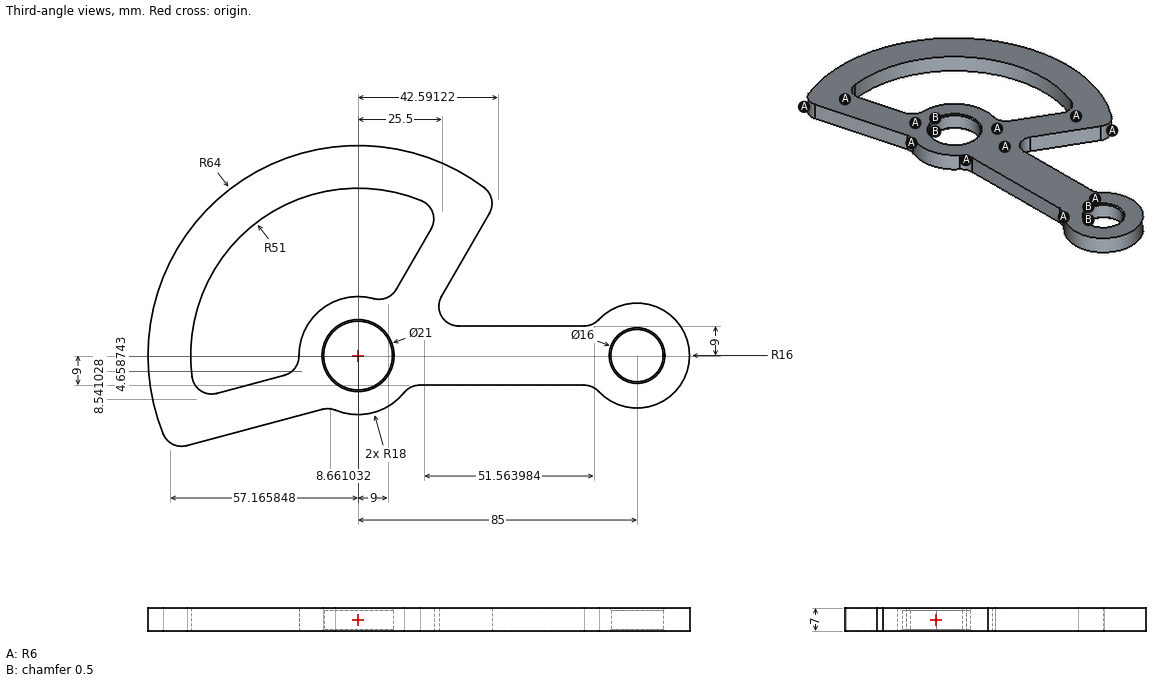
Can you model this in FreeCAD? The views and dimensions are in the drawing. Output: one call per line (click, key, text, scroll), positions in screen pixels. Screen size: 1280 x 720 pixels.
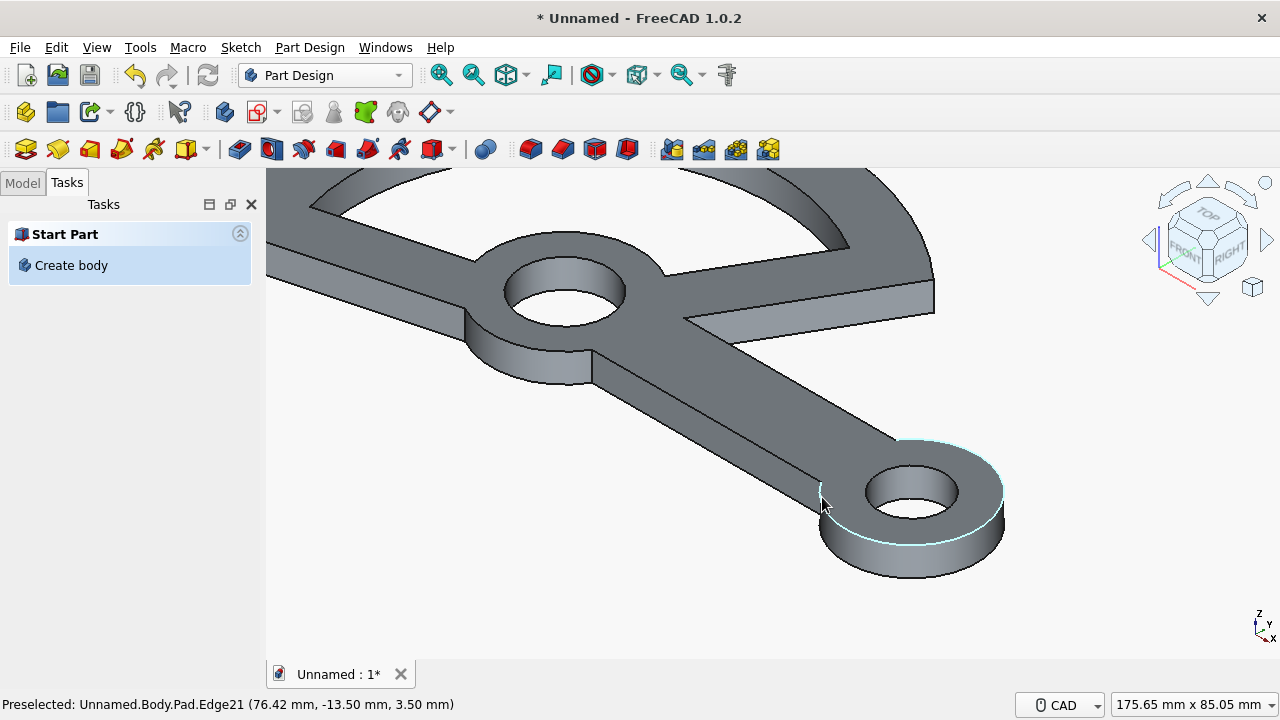
click(442, 76)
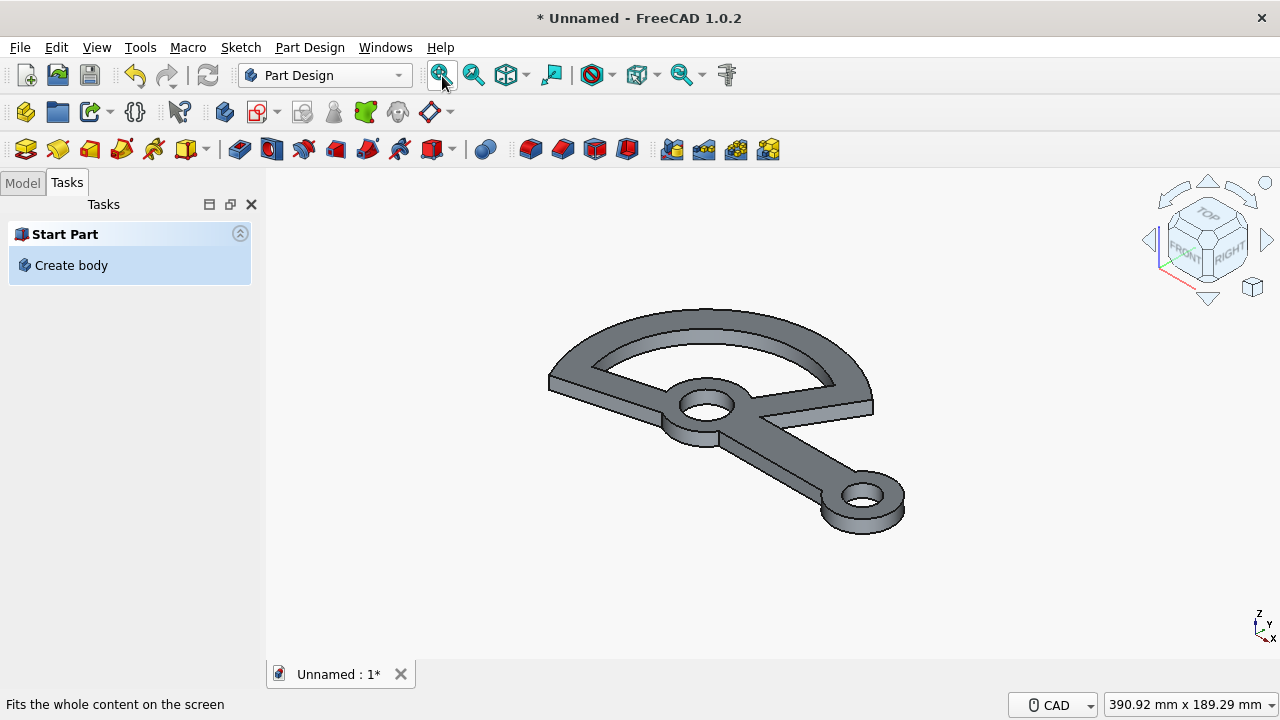
key(2)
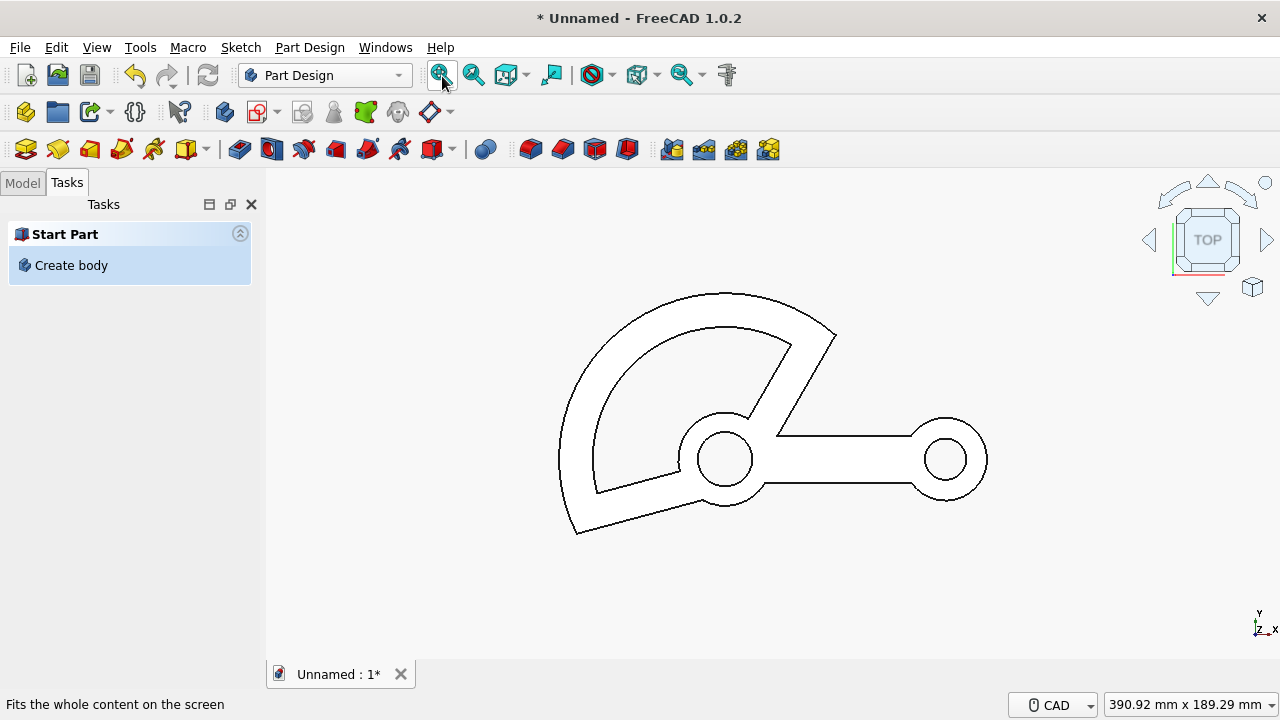
scroll(911, 482, up, 4)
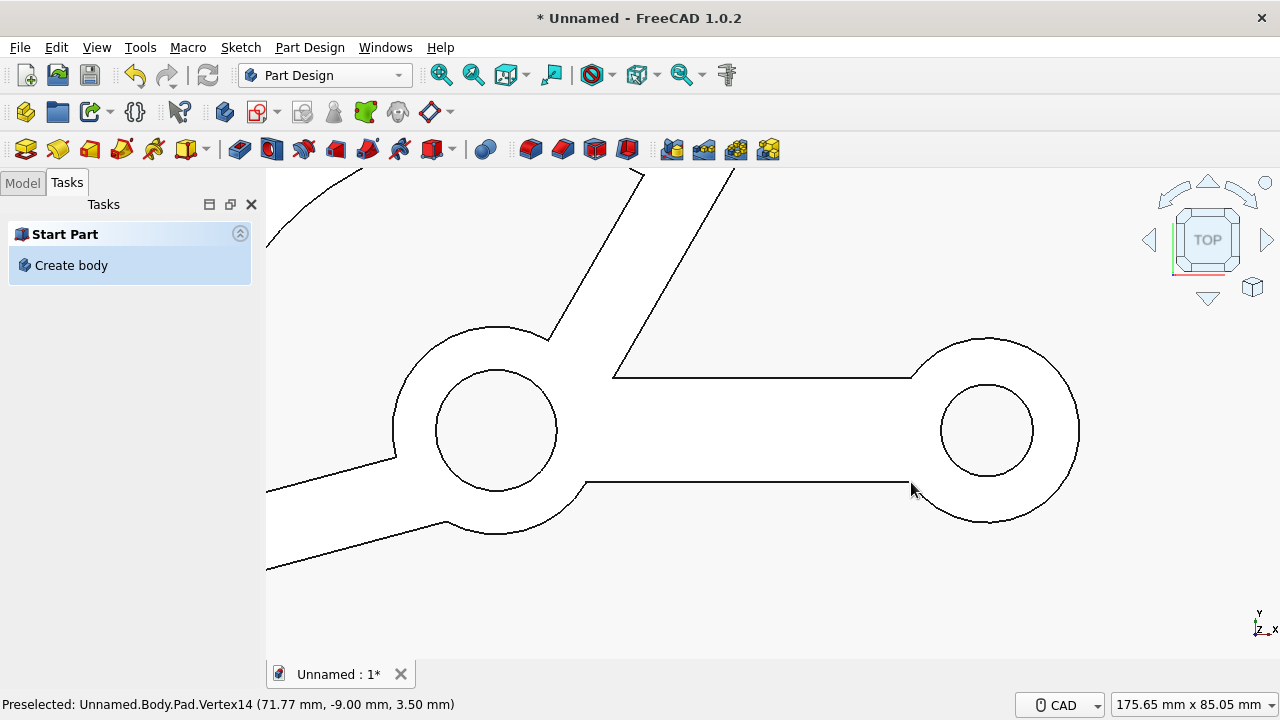
click(442, 76)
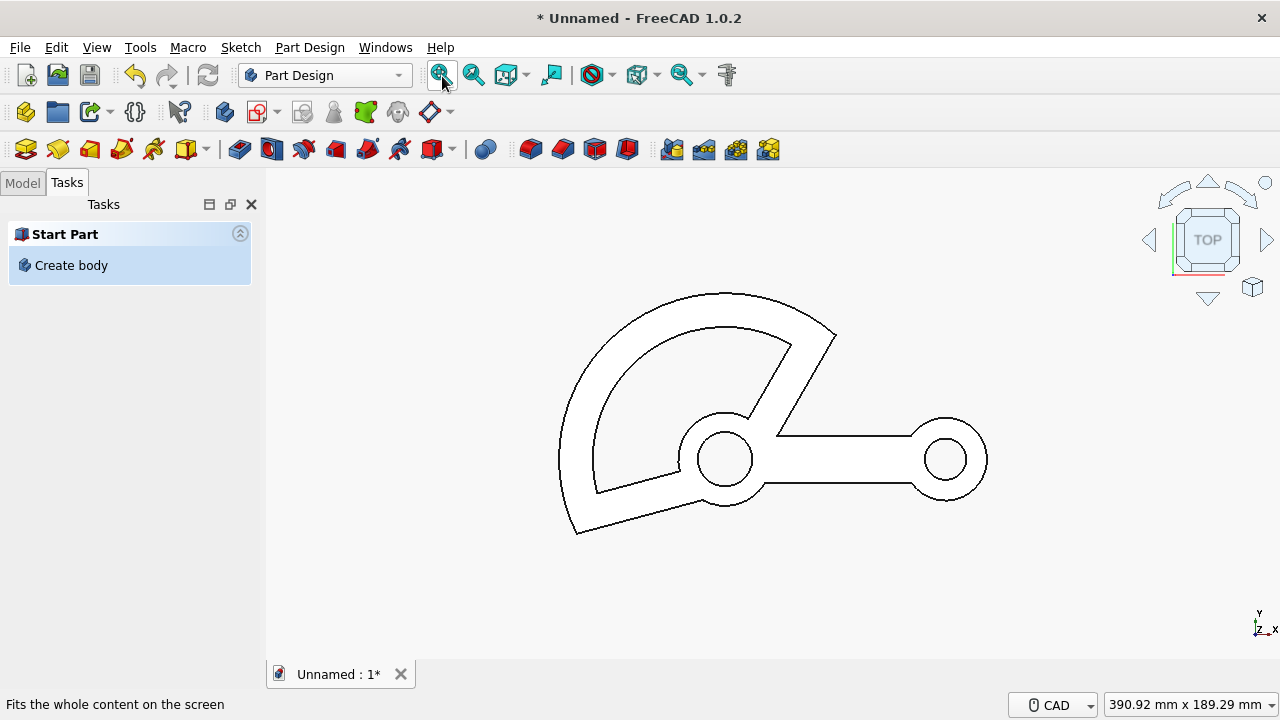
key(1)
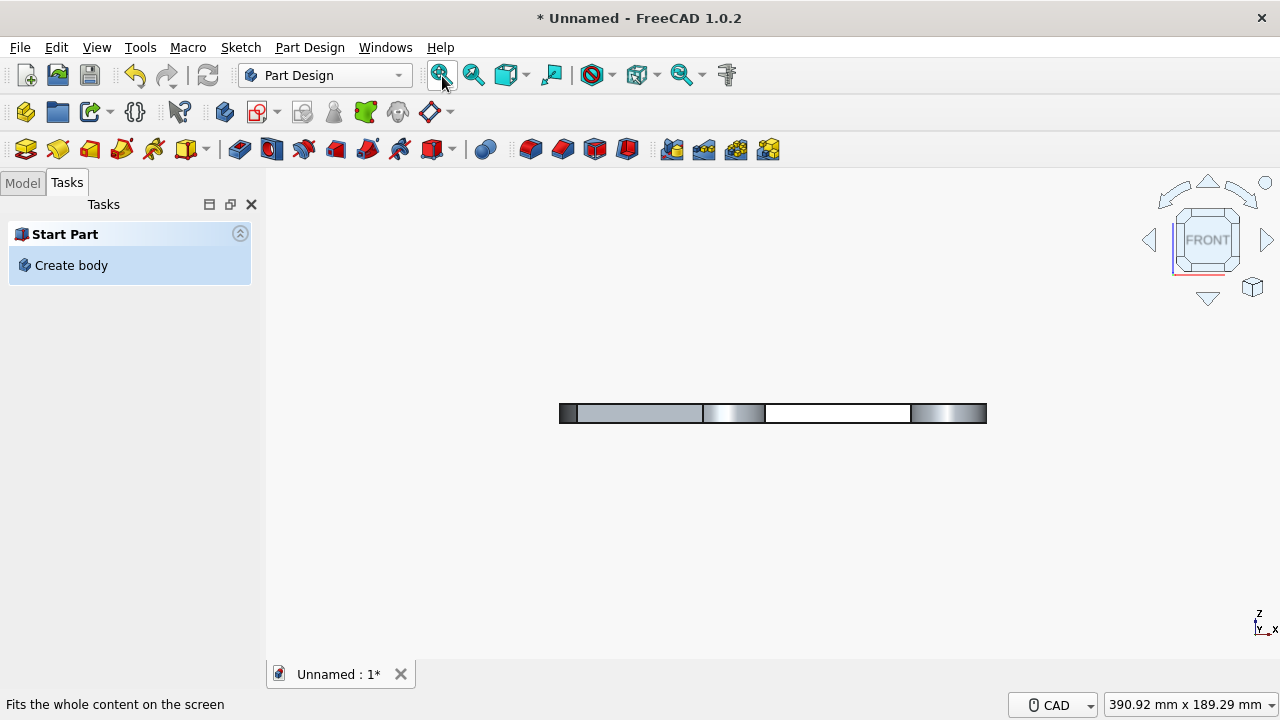
click(442, 76)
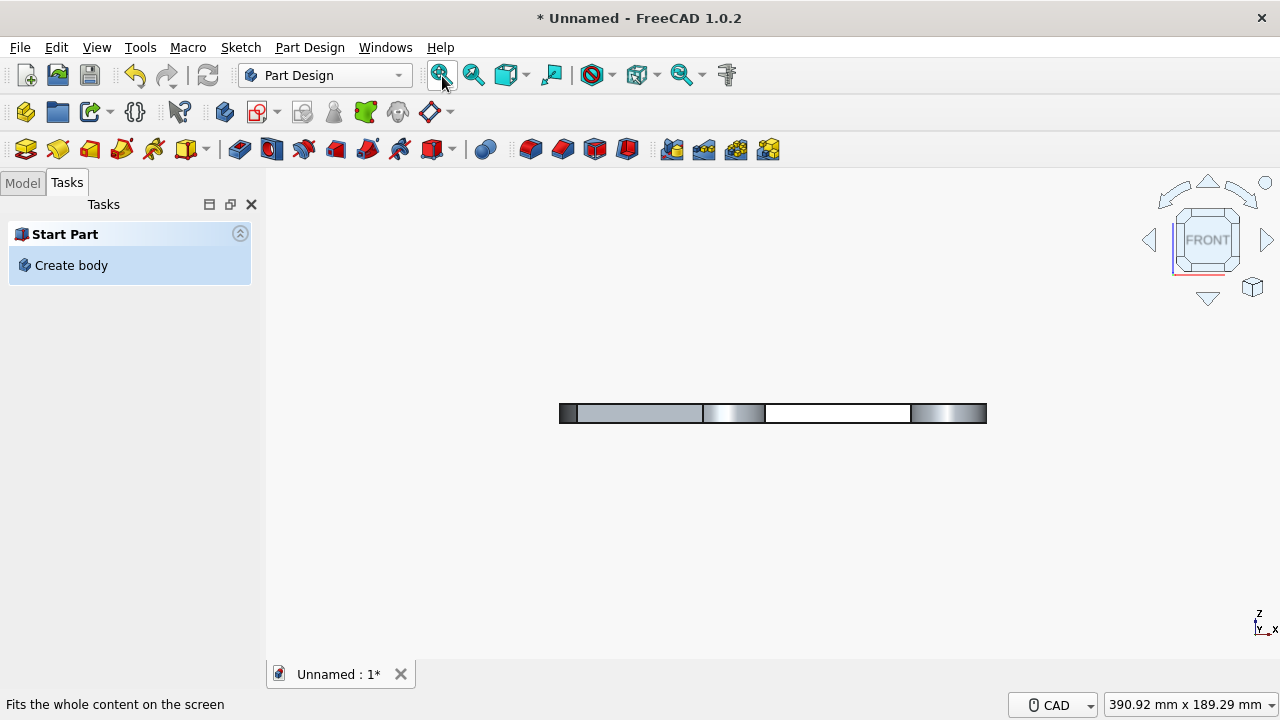
click(577, 413)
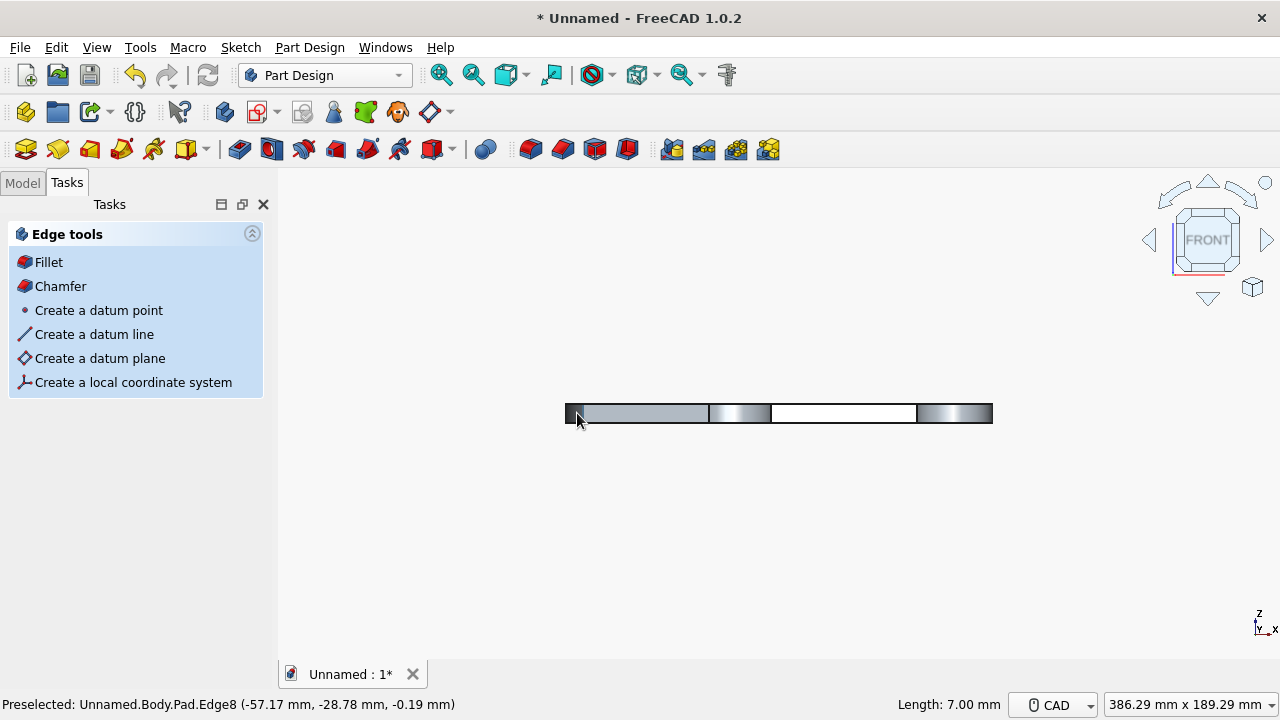
scroll(917, 413, up, 4)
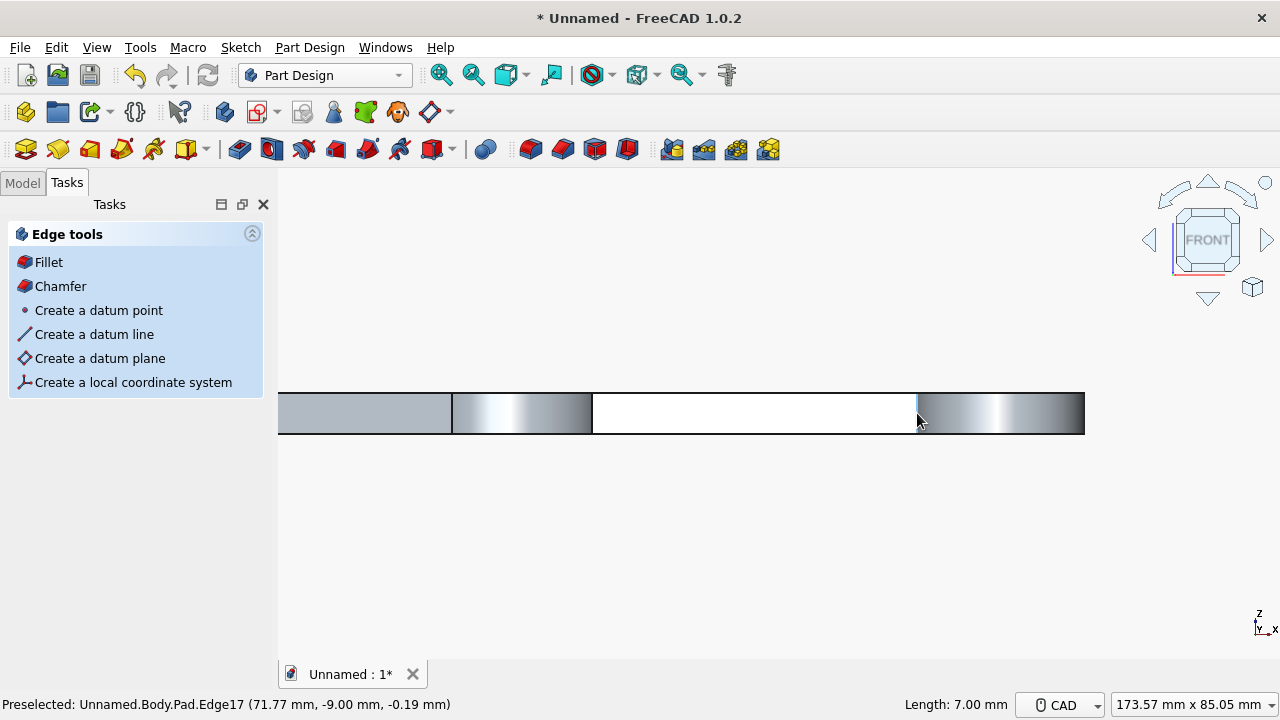
click(442, 76)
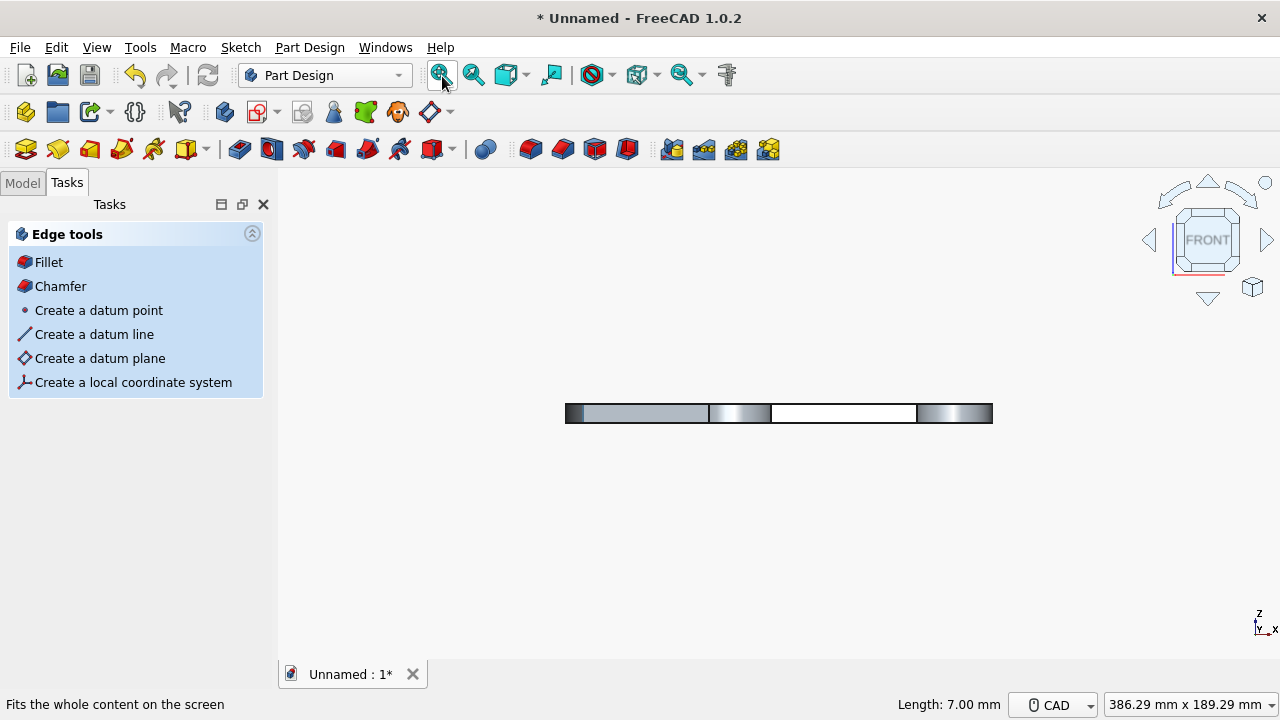
key(3)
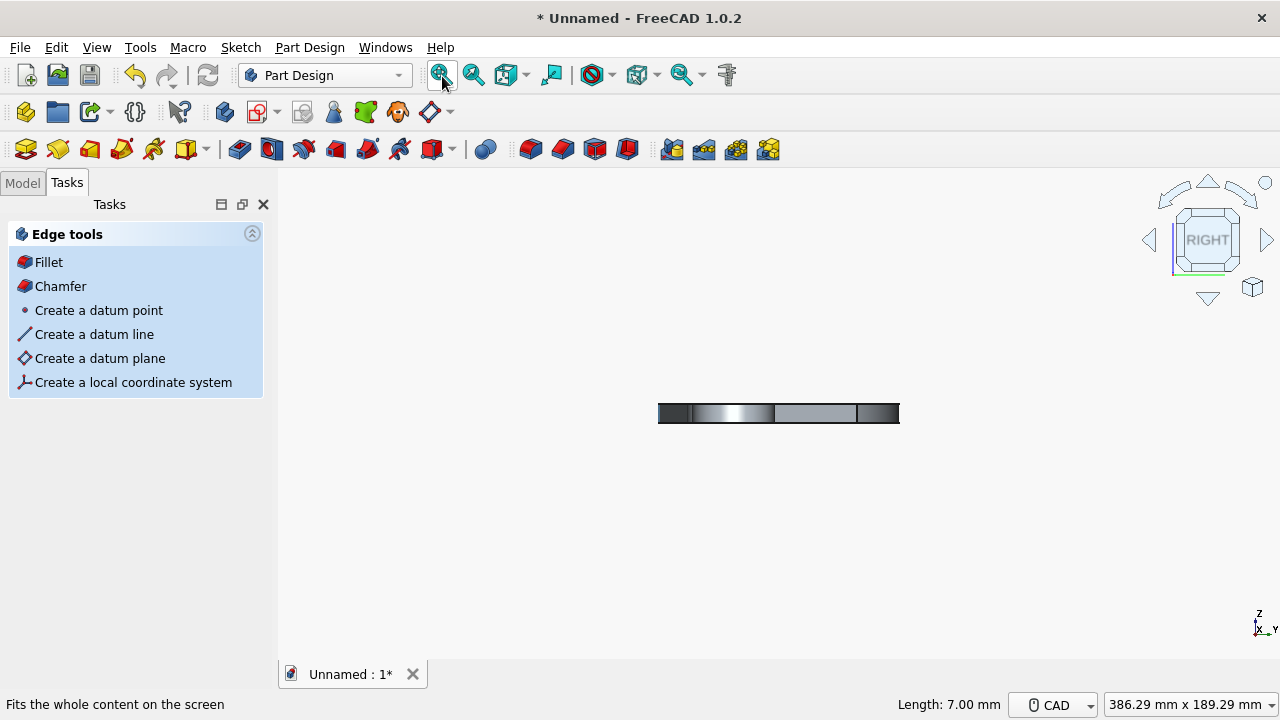
click(442, 76)